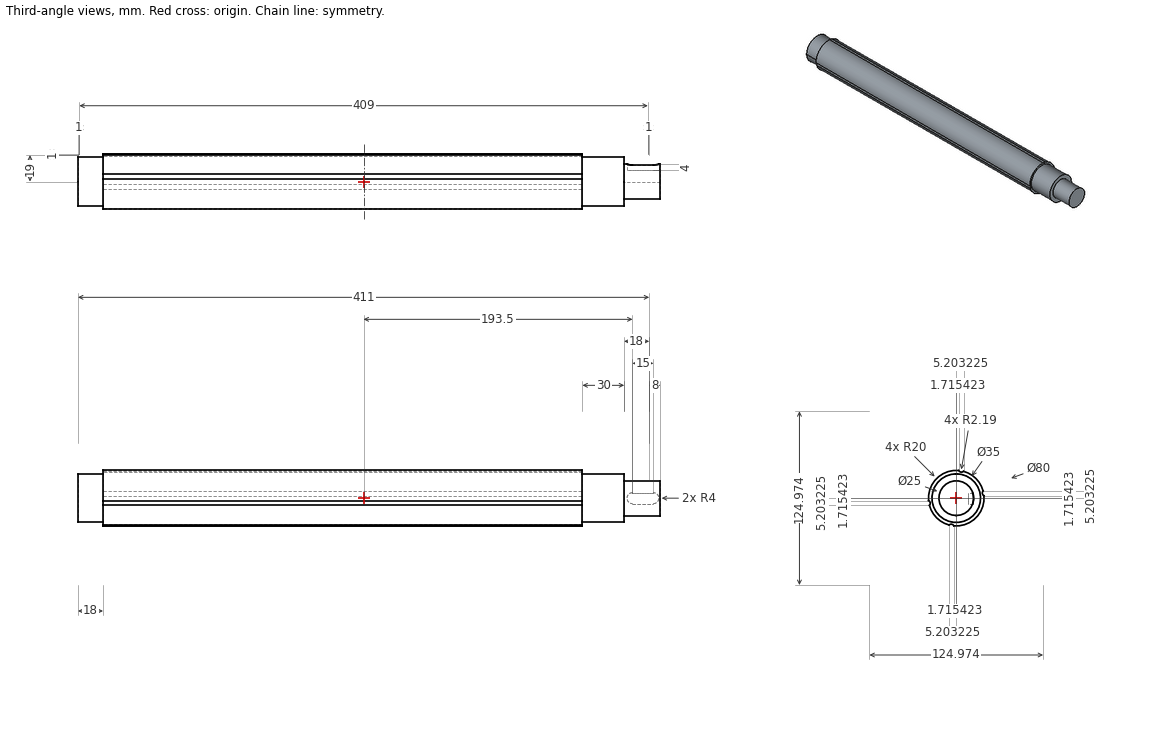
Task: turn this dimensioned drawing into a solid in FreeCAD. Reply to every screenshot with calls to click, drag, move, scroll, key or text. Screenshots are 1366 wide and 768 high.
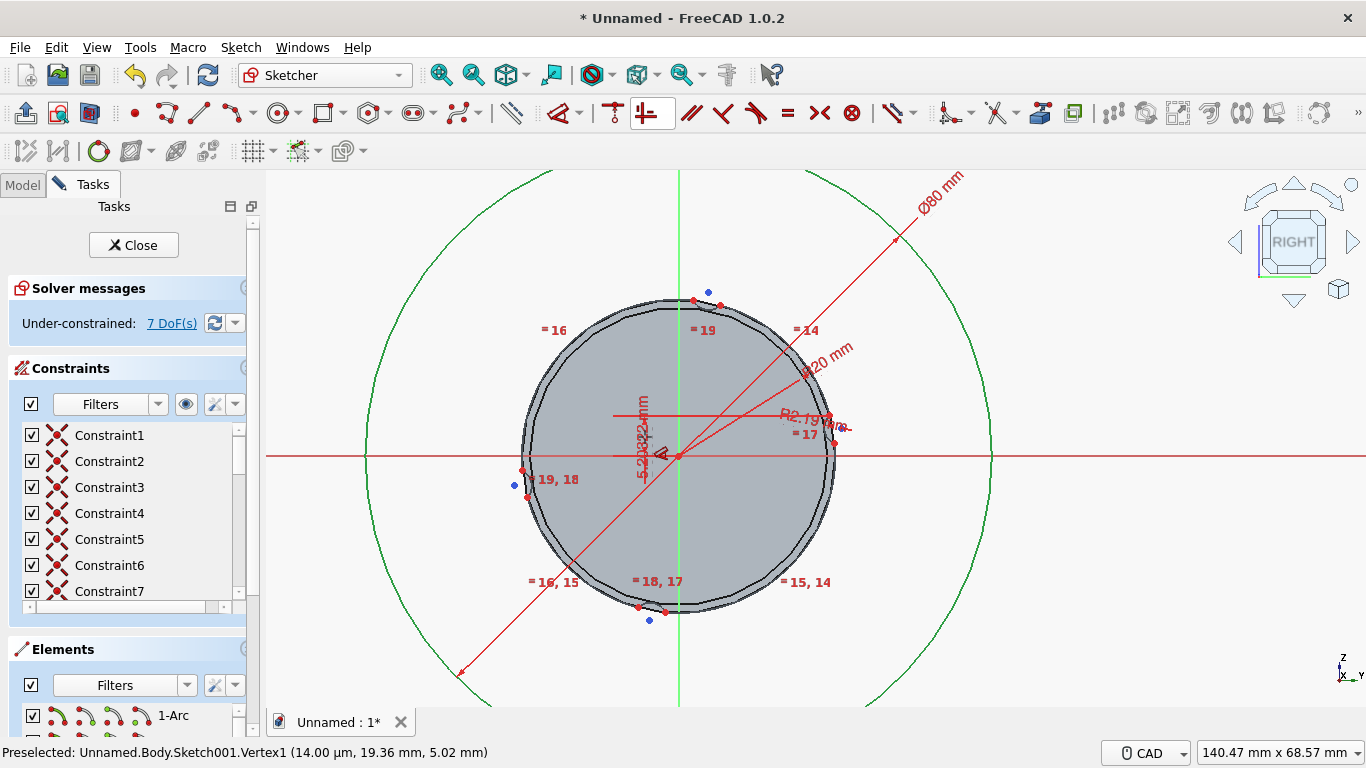
click(720, 305)
click(699, 271)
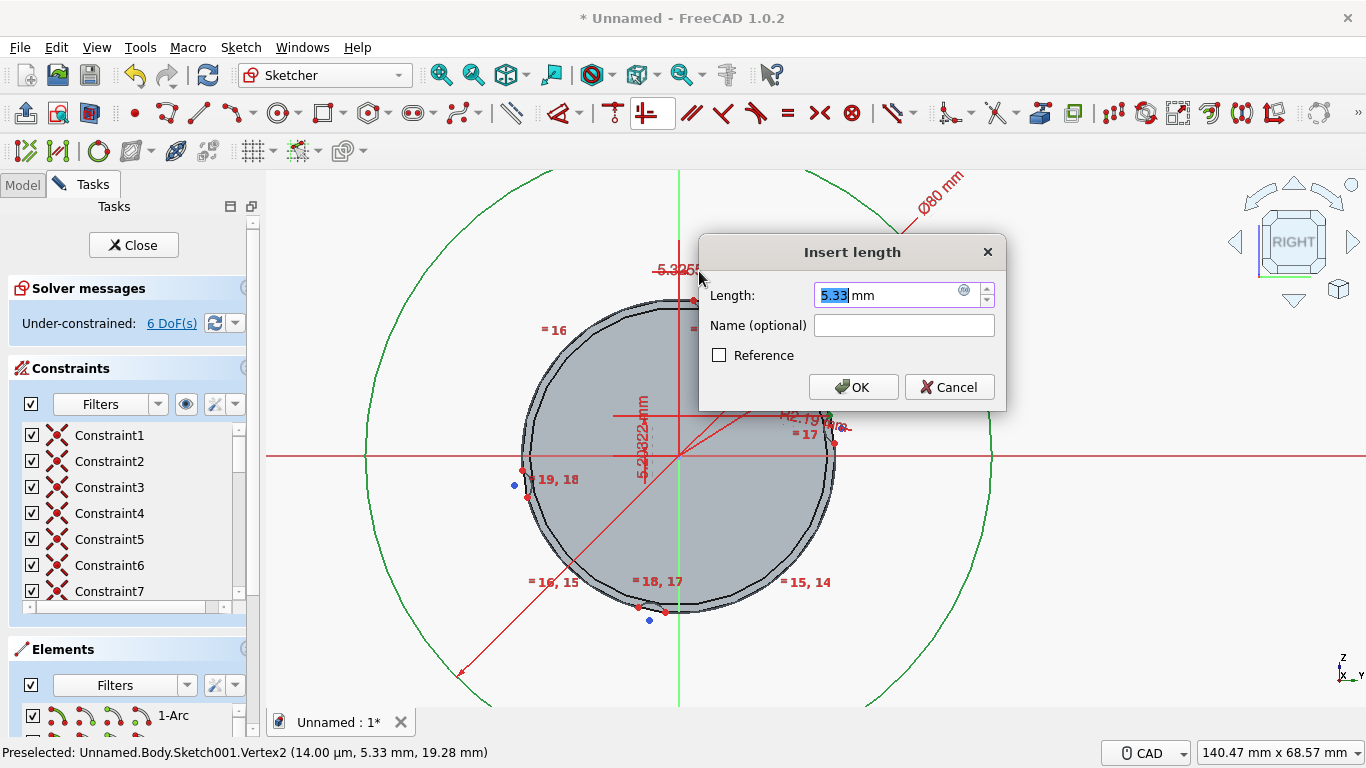
text(5.203225)
key(Return)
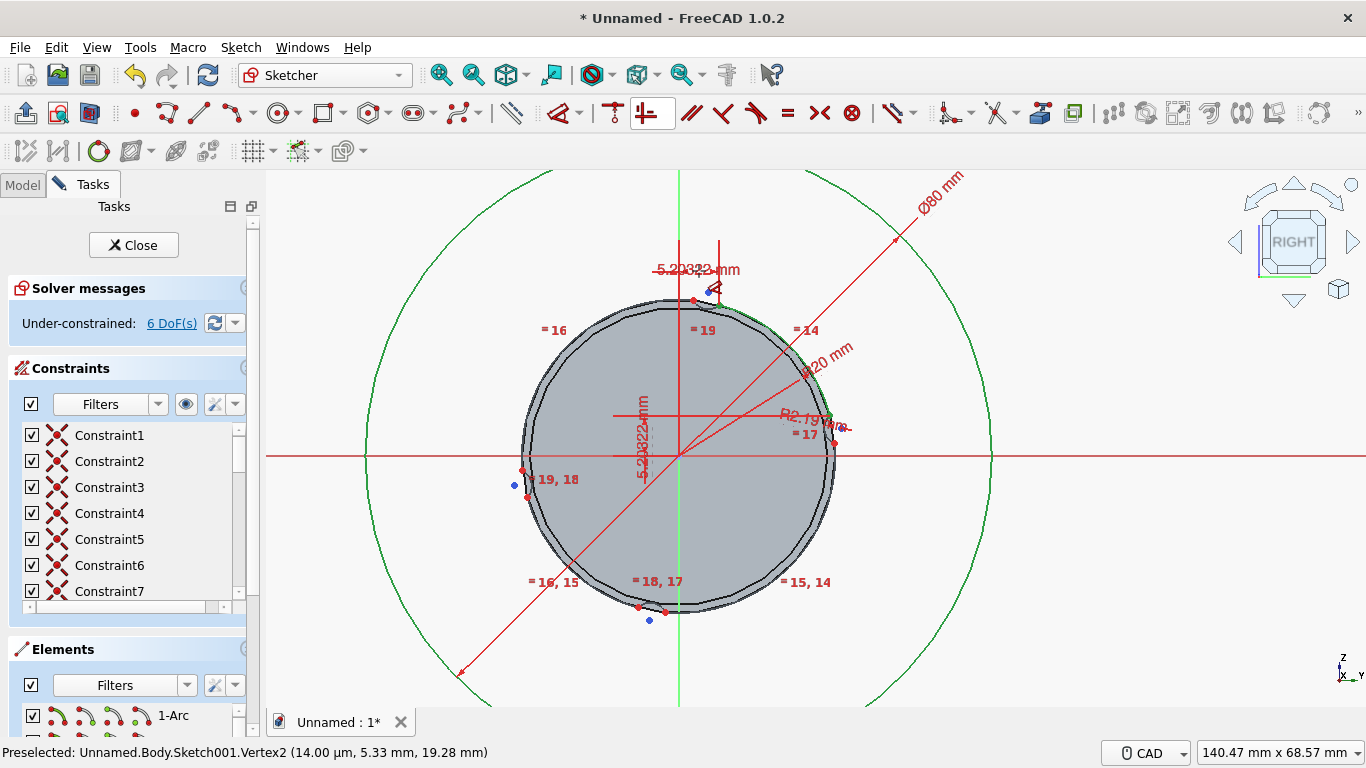
scroll(835, 444, up, 6)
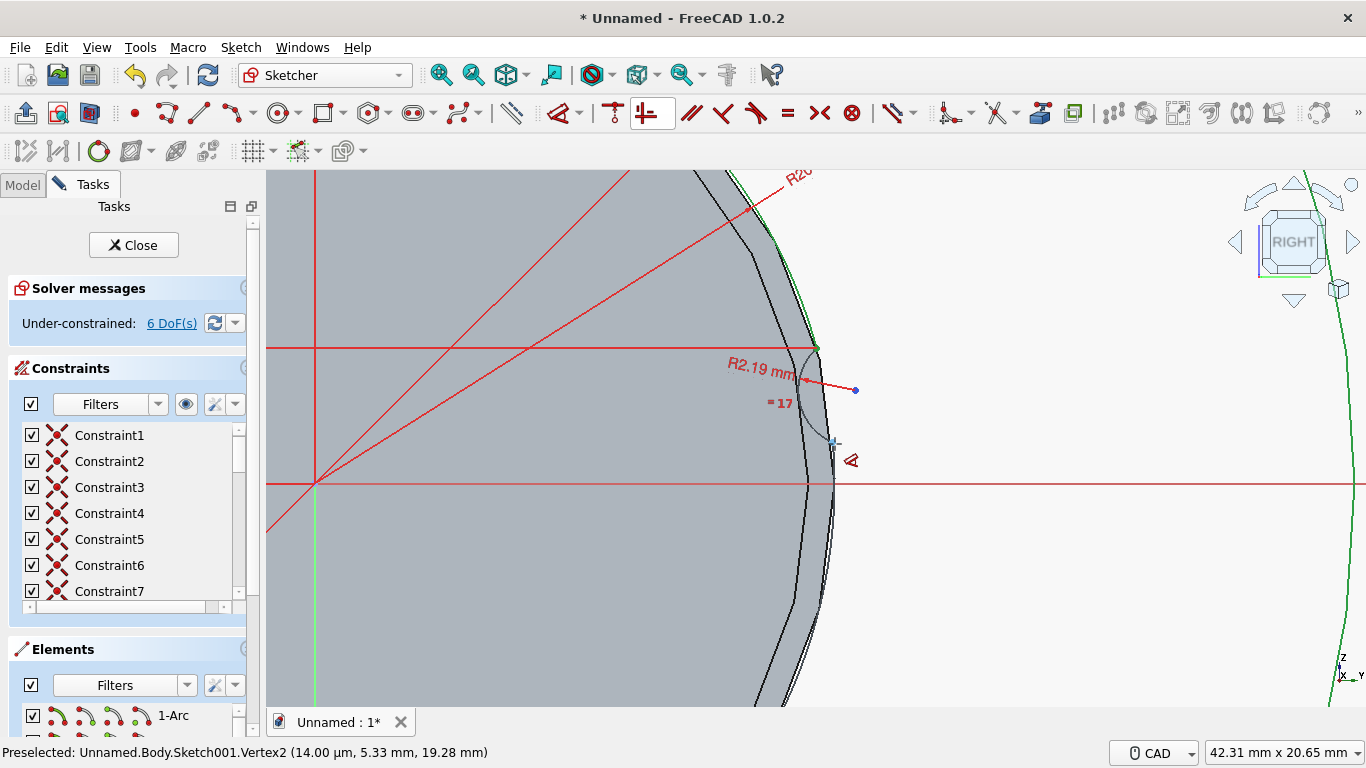
click(833, 443)
click(867, 463)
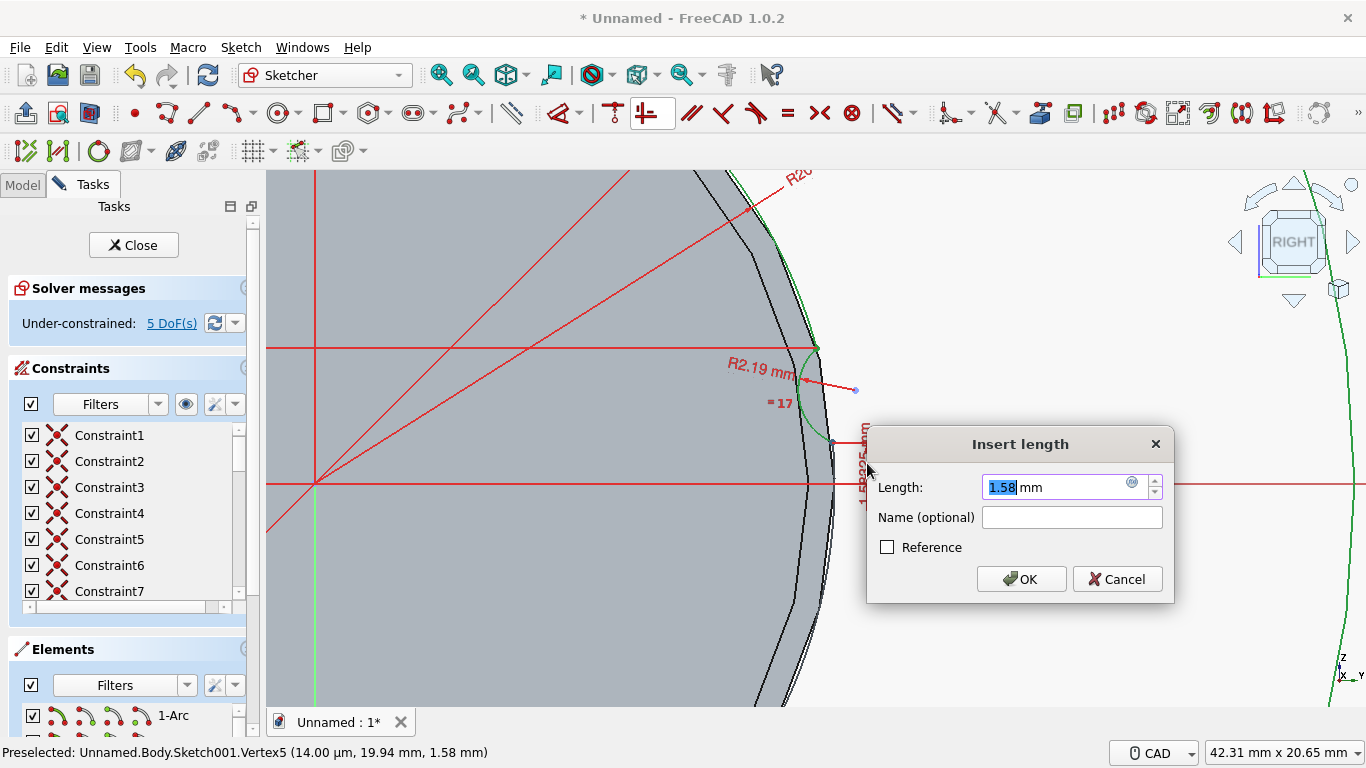
text(1.715423)
key(Return)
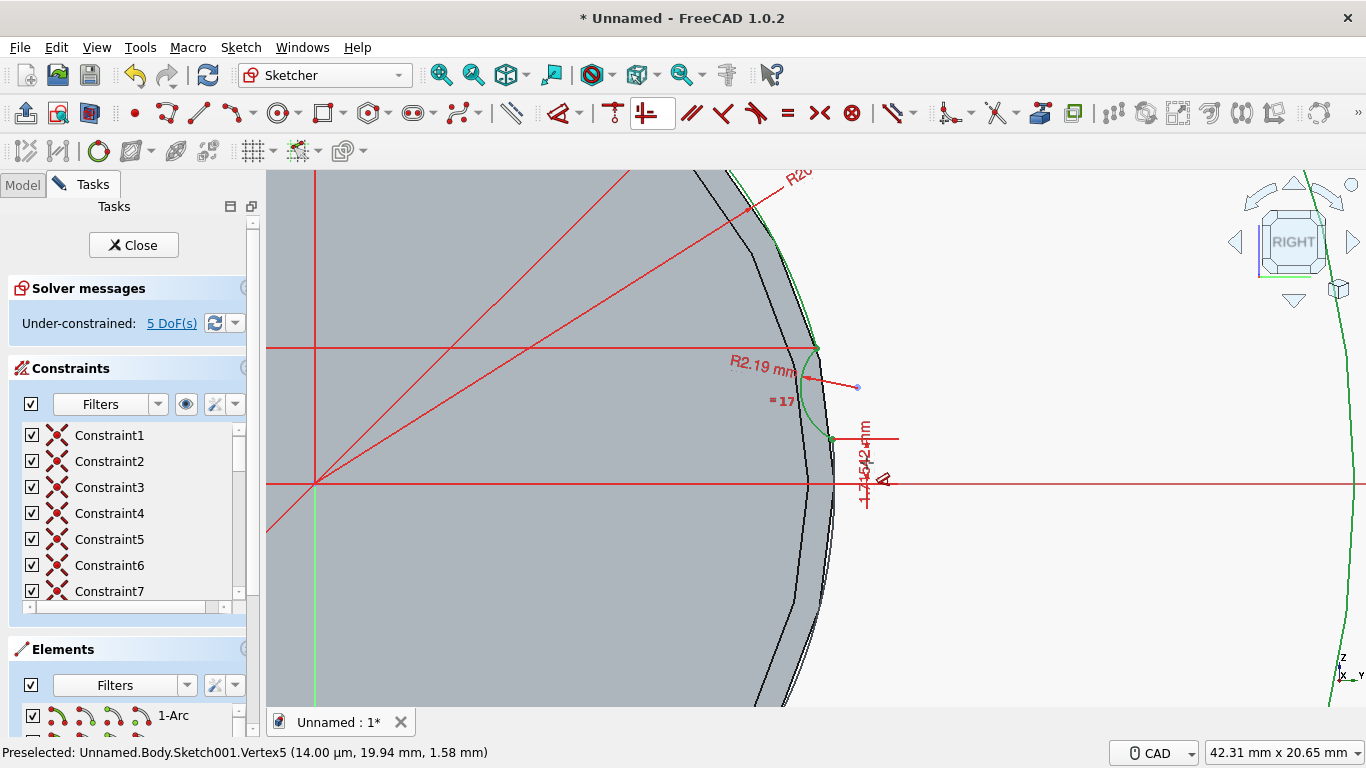
scroll(833, 430, down, 9)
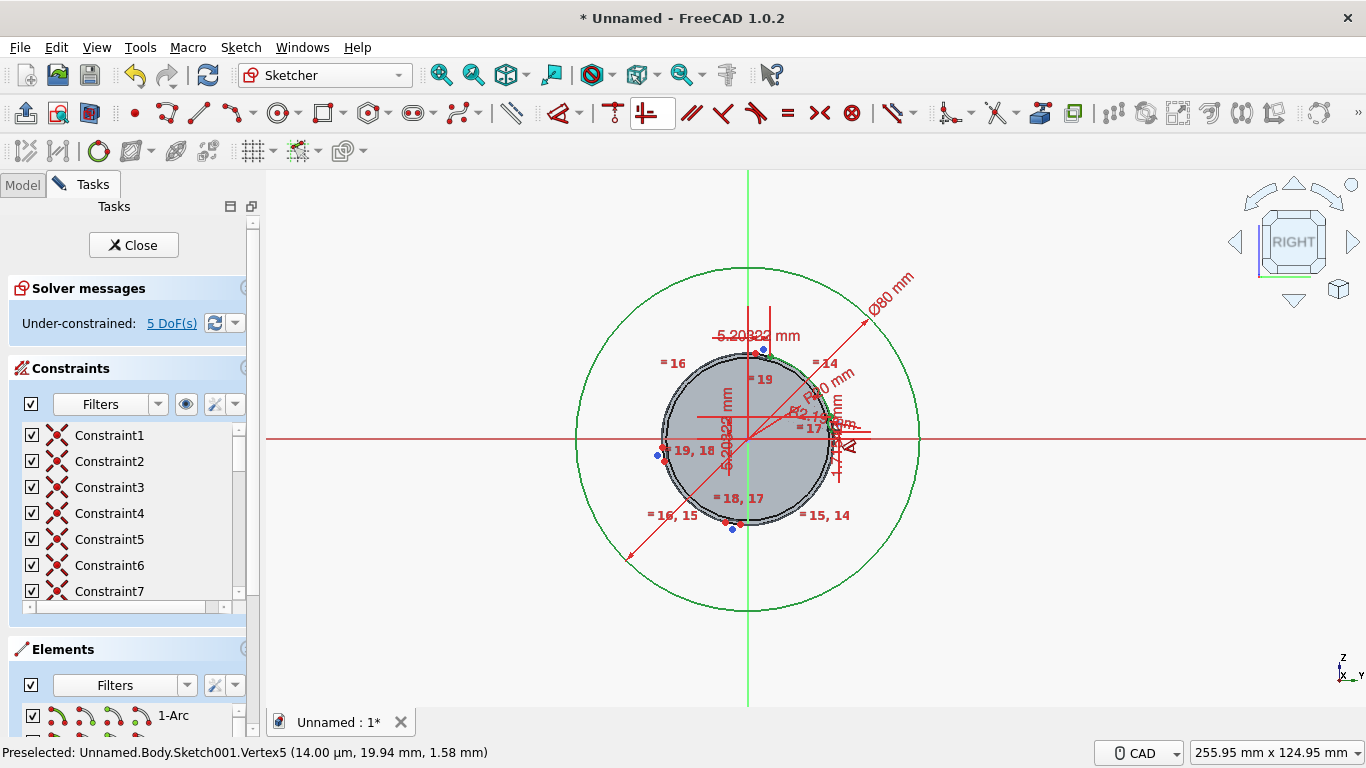
scroll(740, 525, up, 9)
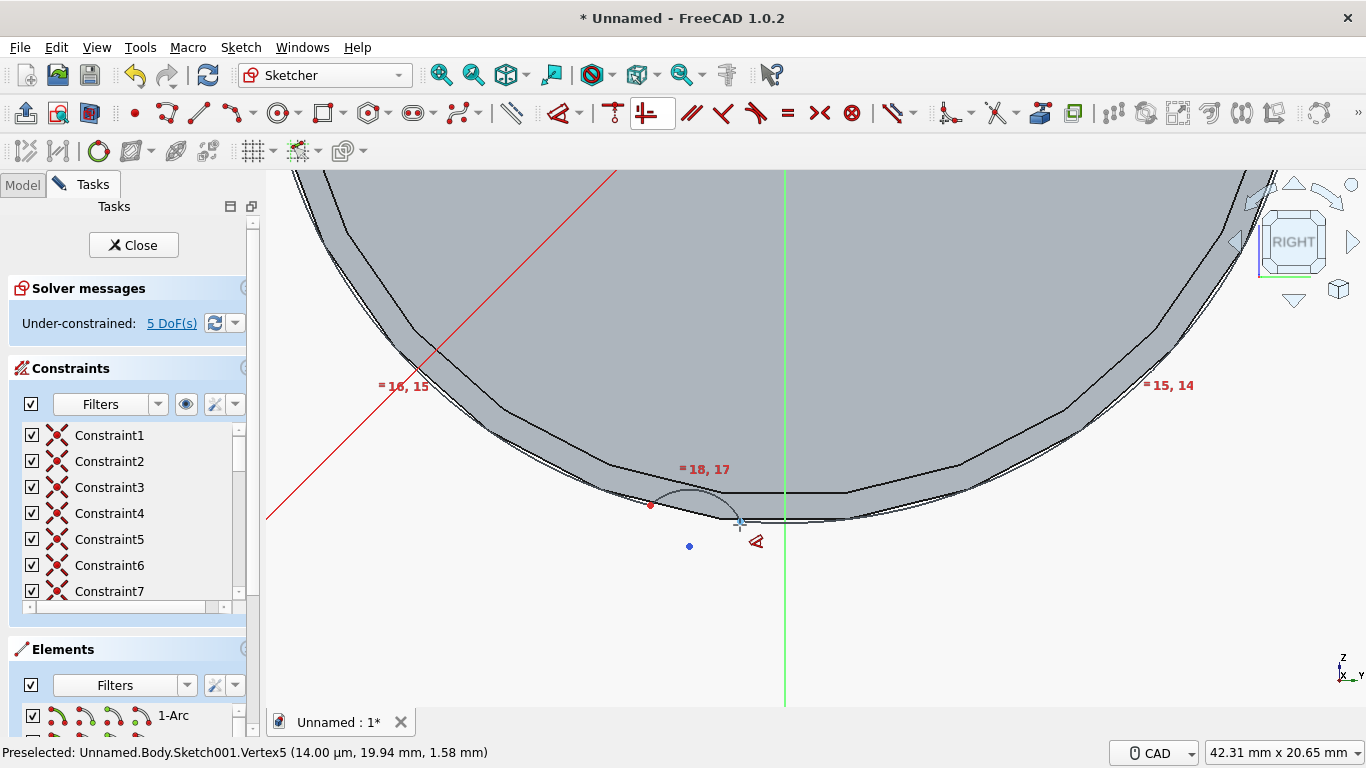
click(741, 521)
click(763, 555)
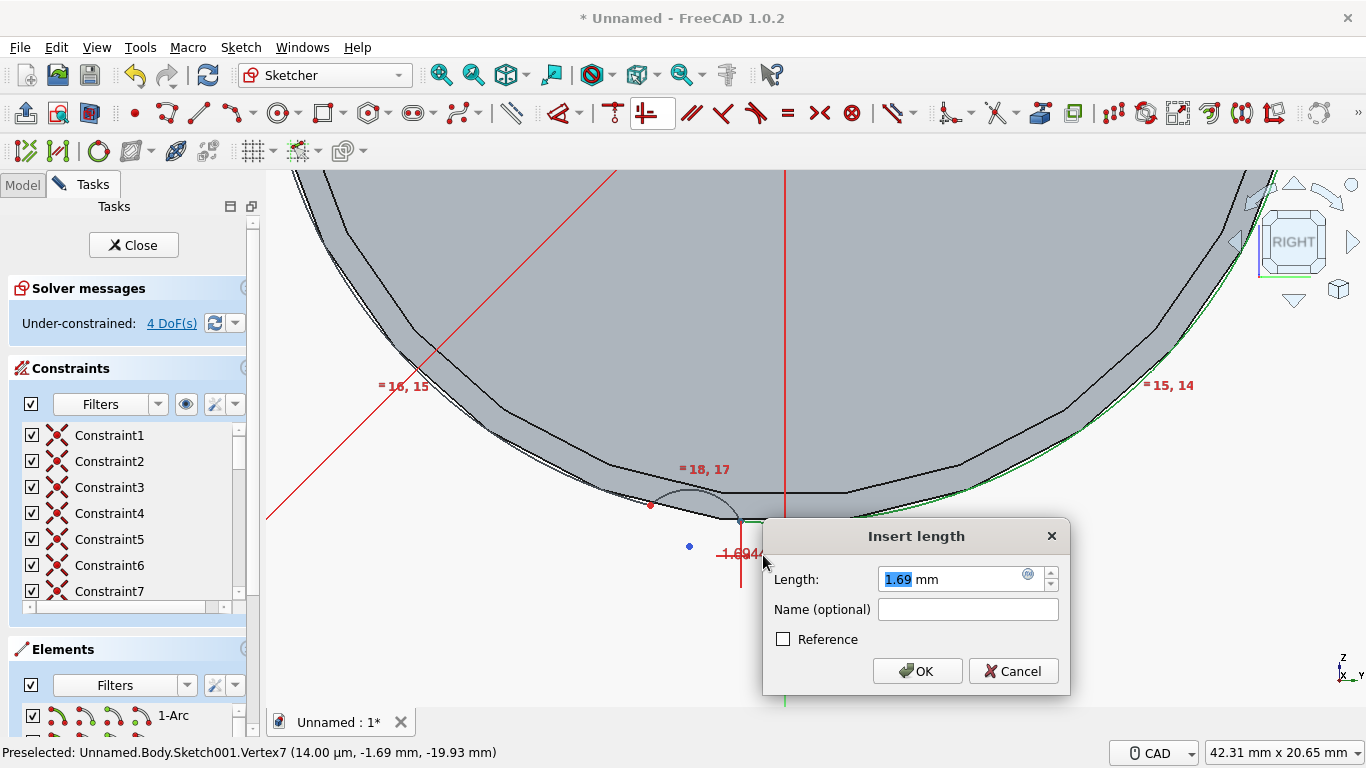
text(1.715423)
key(Return)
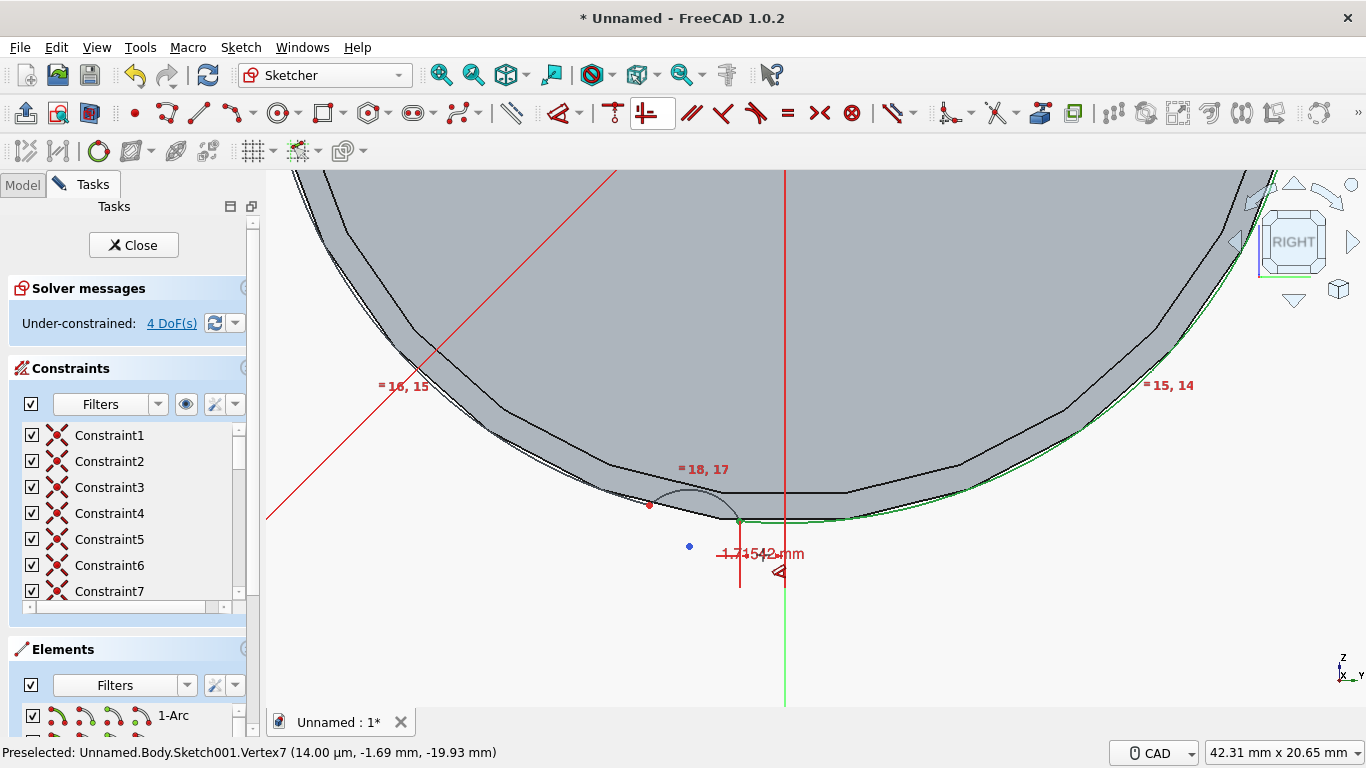
scroll(740, 525, down, 9)